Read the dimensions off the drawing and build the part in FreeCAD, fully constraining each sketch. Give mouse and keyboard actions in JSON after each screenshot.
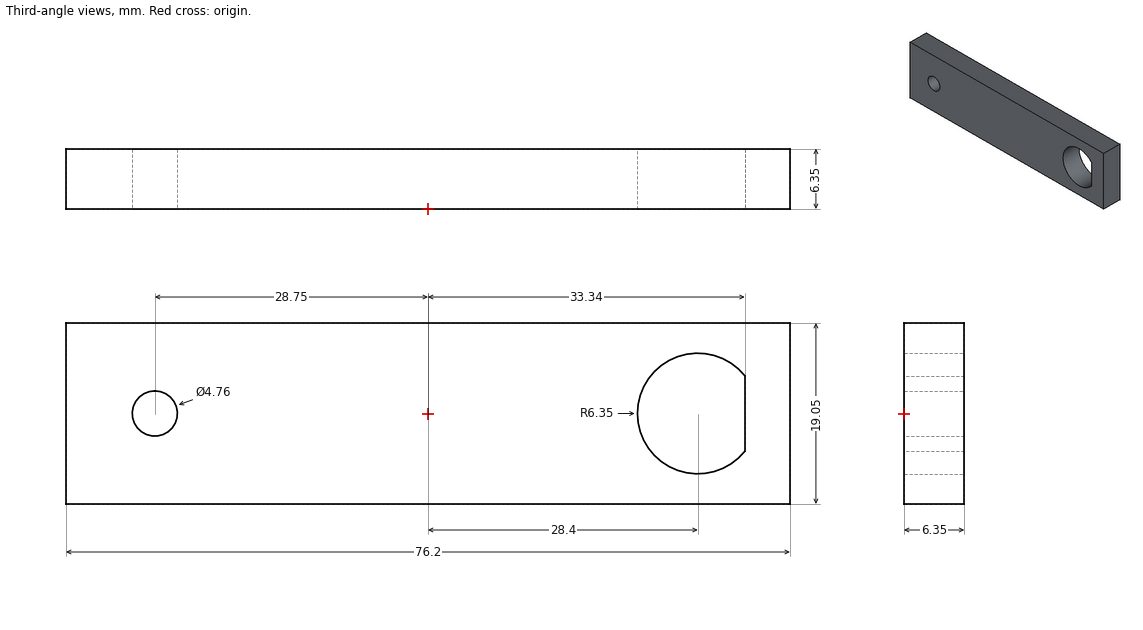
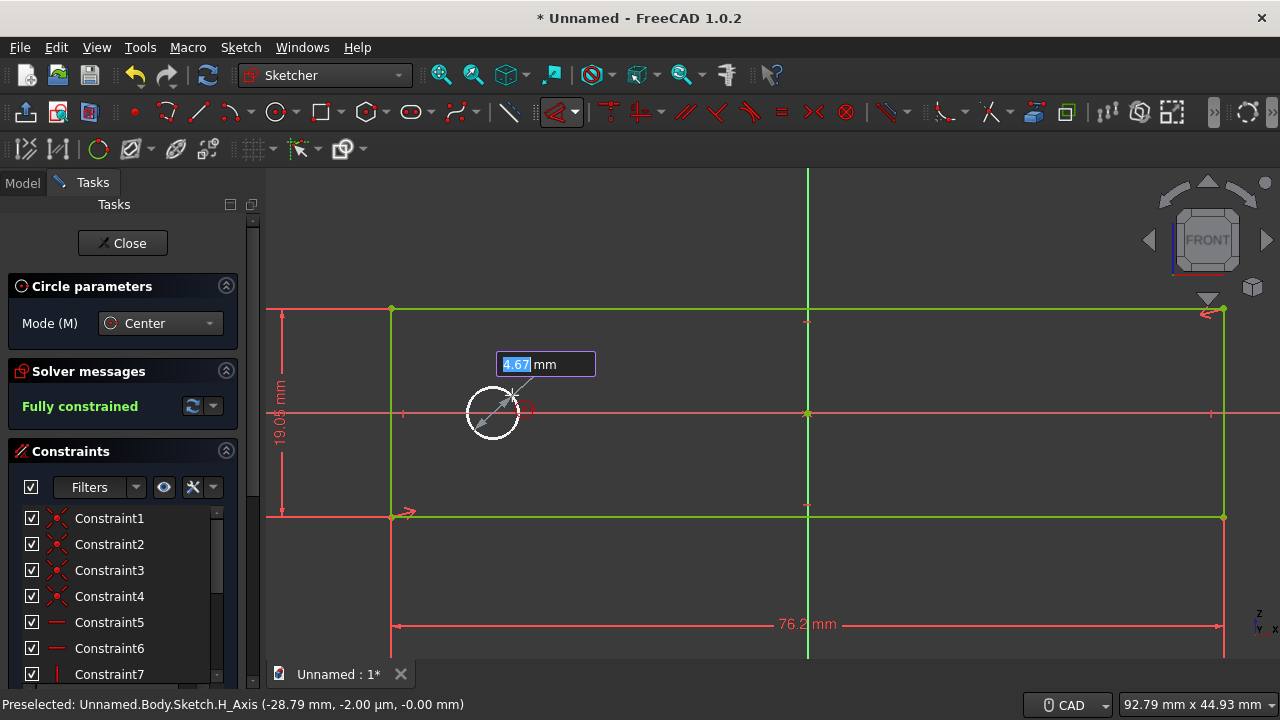
{"action": "type", "text": "4.76"}
{"action": "key", "text": "Return"}
{"action": "key", "text": "Escape"}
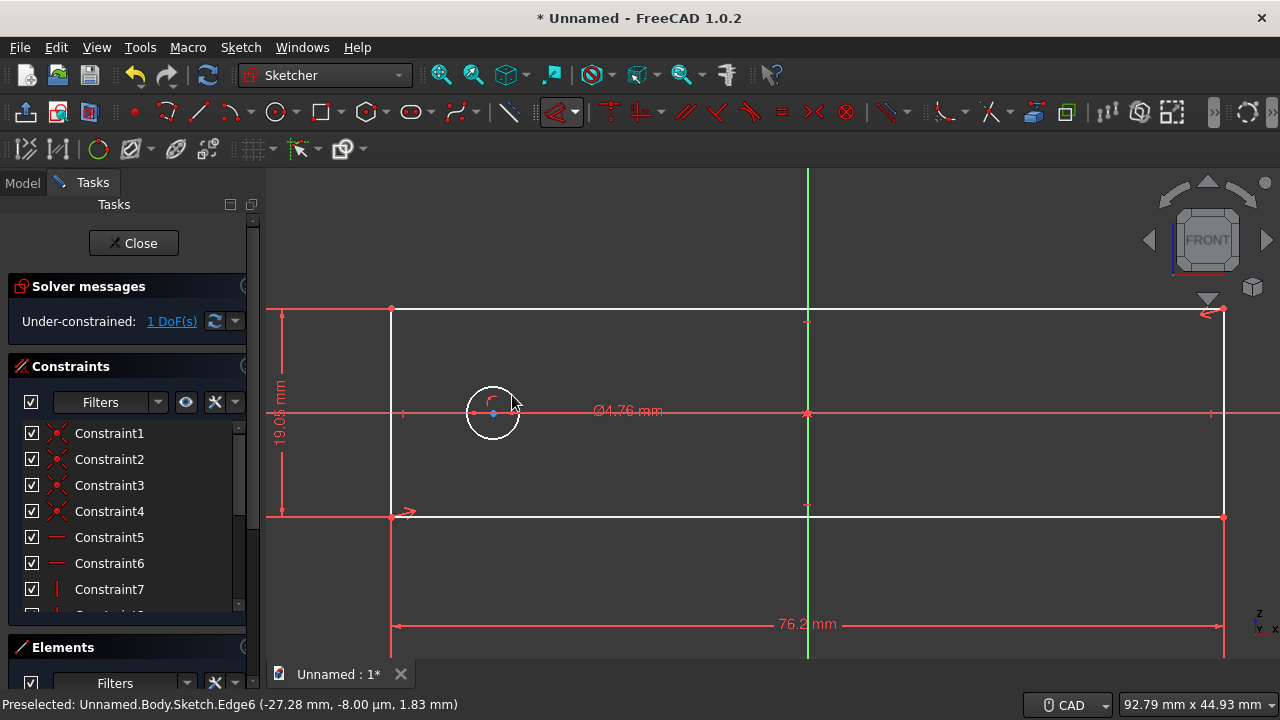
{"action": "left_click", "coordinate": [493, 413]}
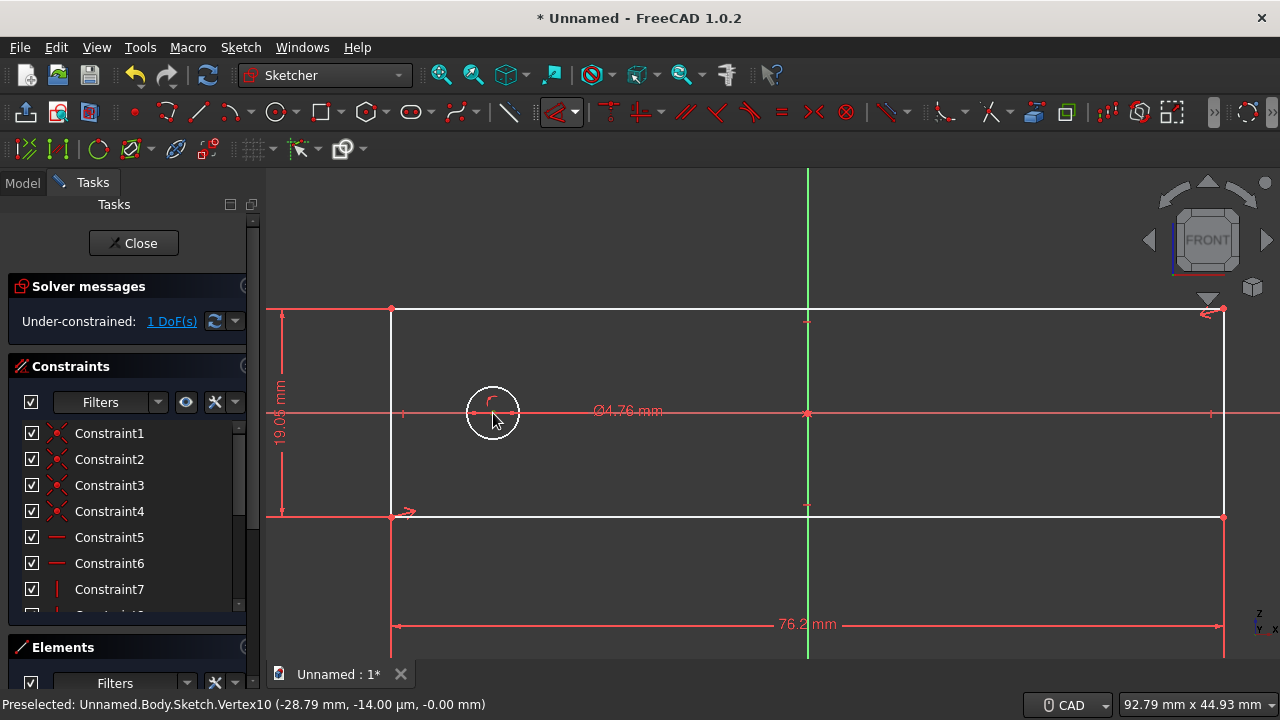
{"action": "left_click", "coordinate": [578, 112]}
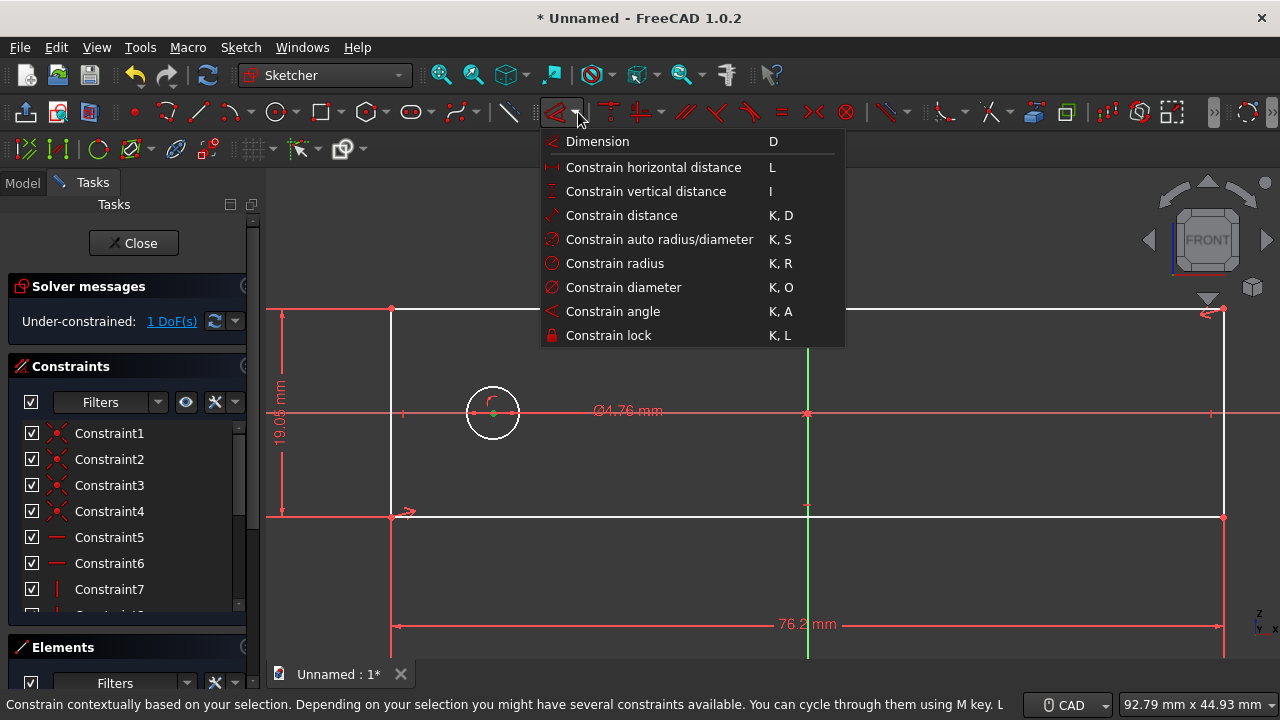
{"action": "left_click", "coordinate": [693, 167]}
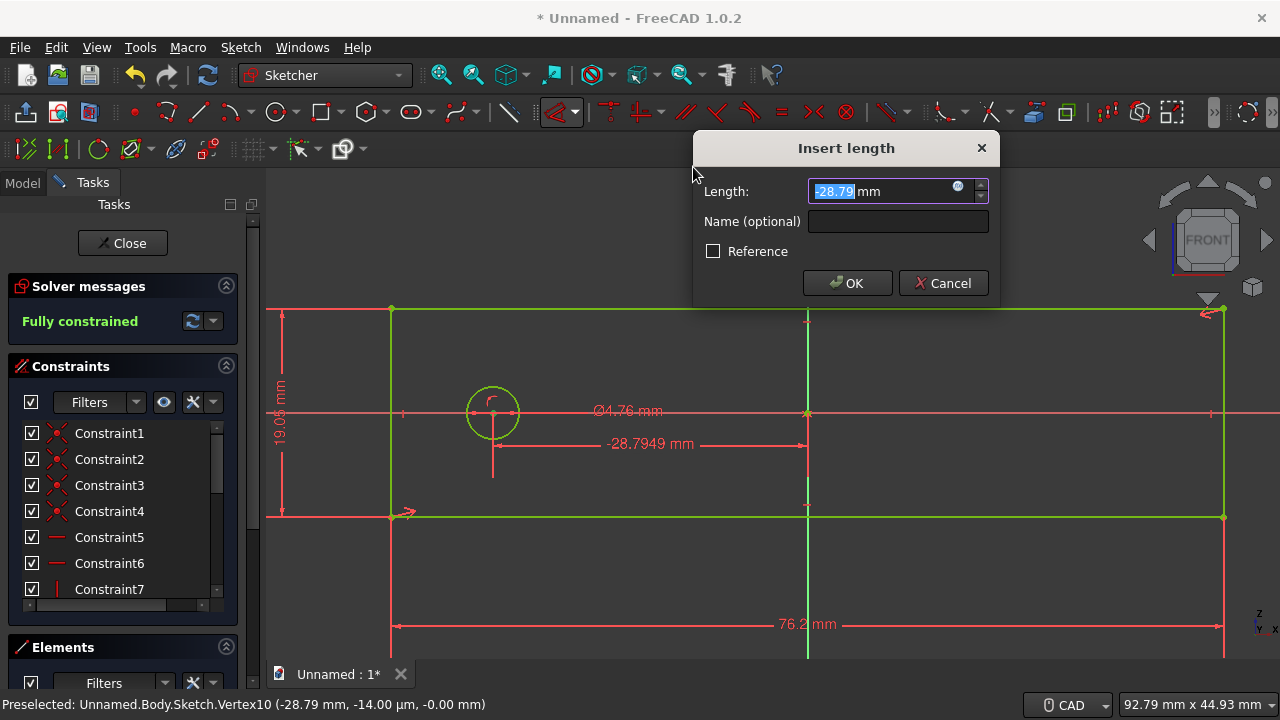
{"action": "type", "text": "-28.75"}
{"action": "key", "text": "Return"}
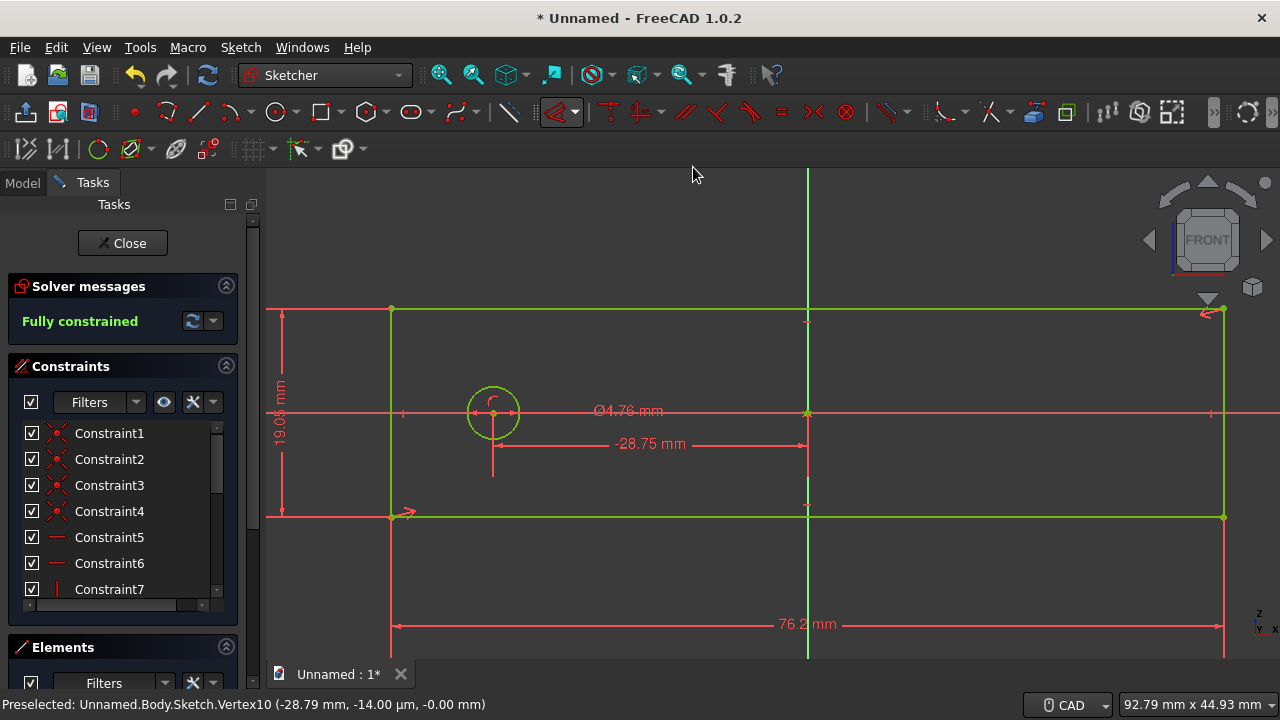
{"action": "left_click", "coordinate": [123, 243]}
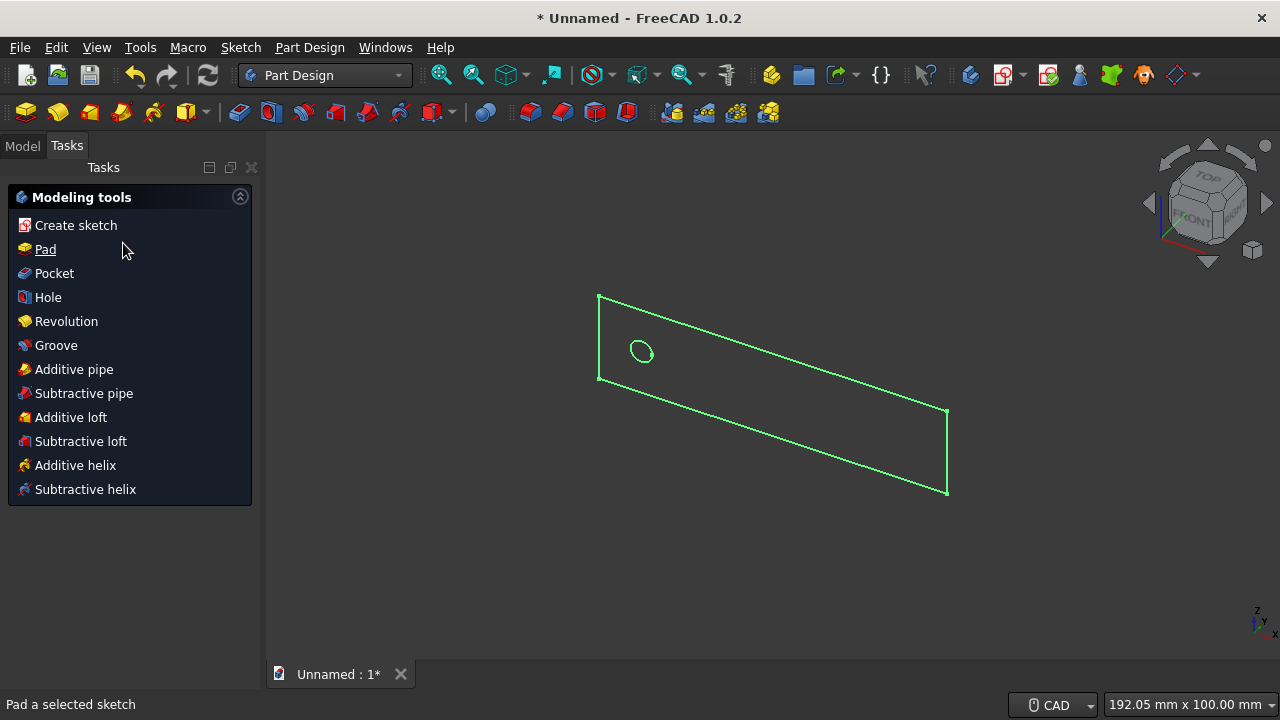
{"action": "left_click", "coordinate": [26, 112]}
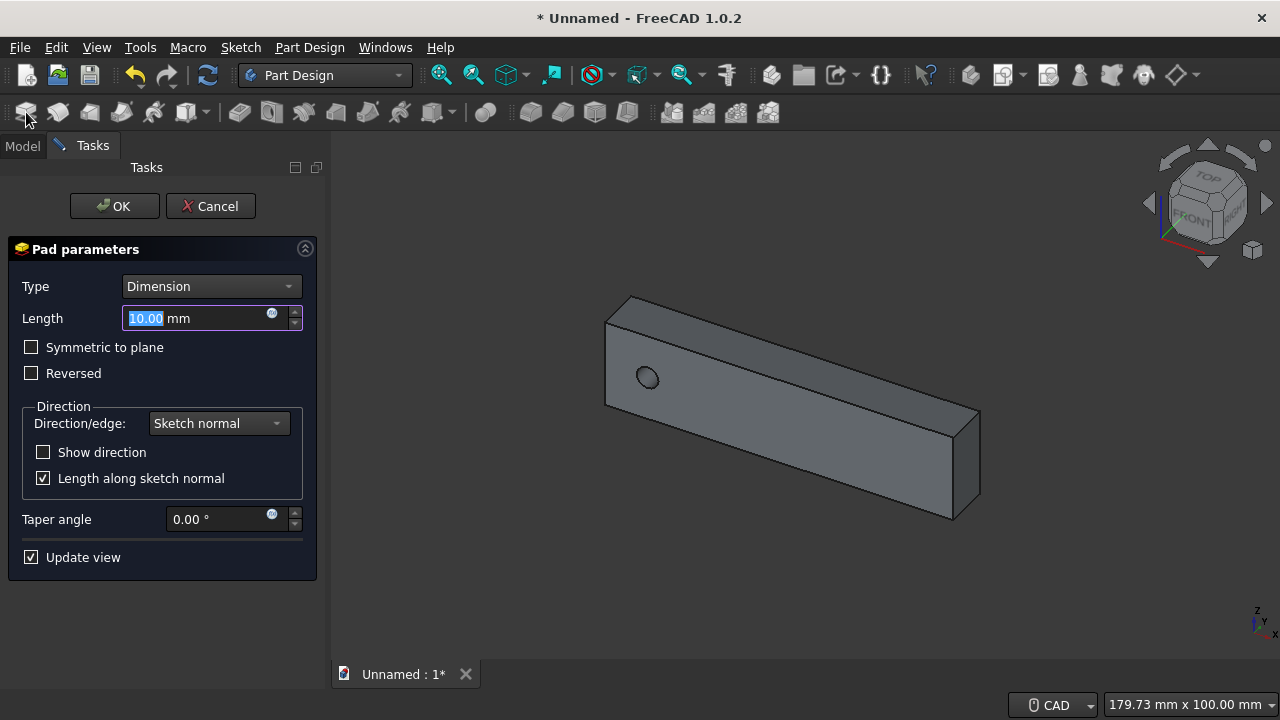
{"action": "type", "text": "6.35"}
{"action": "key", "text": "Tab"}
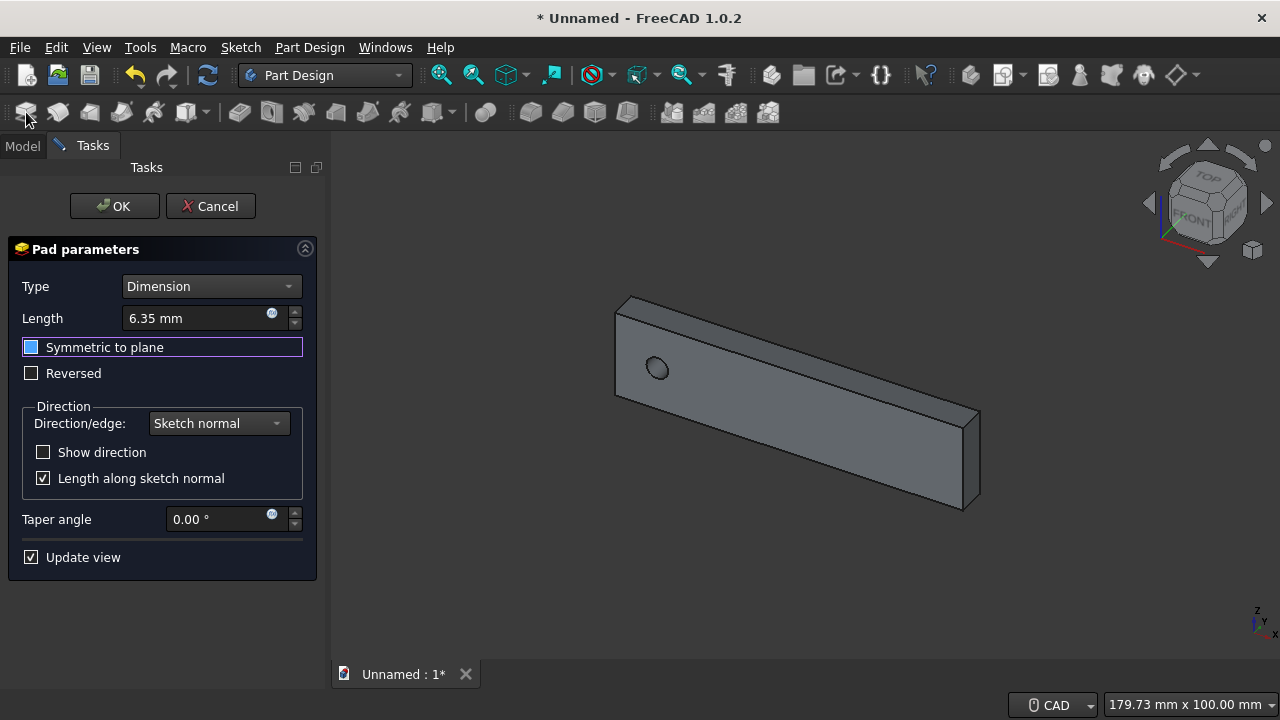
{"action": "left_click", "coordinate": [30, 373]}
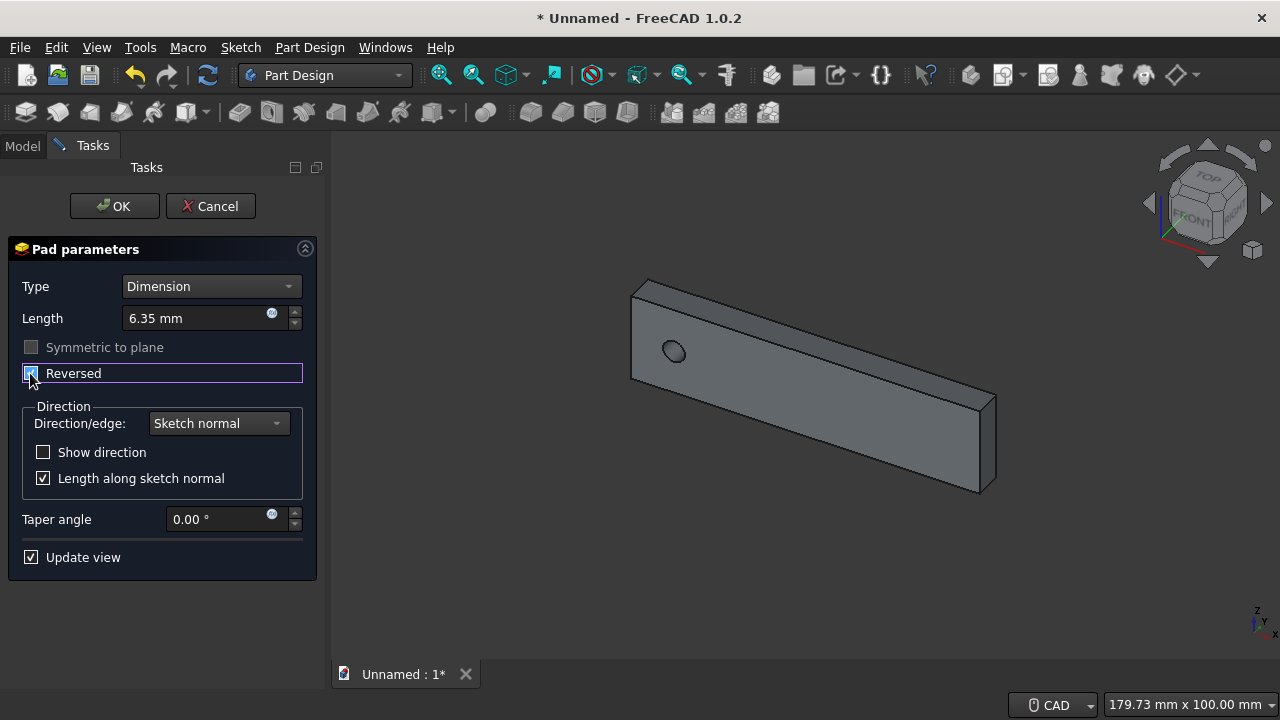
{"action": "left_click", "coordinate": [115, 206]}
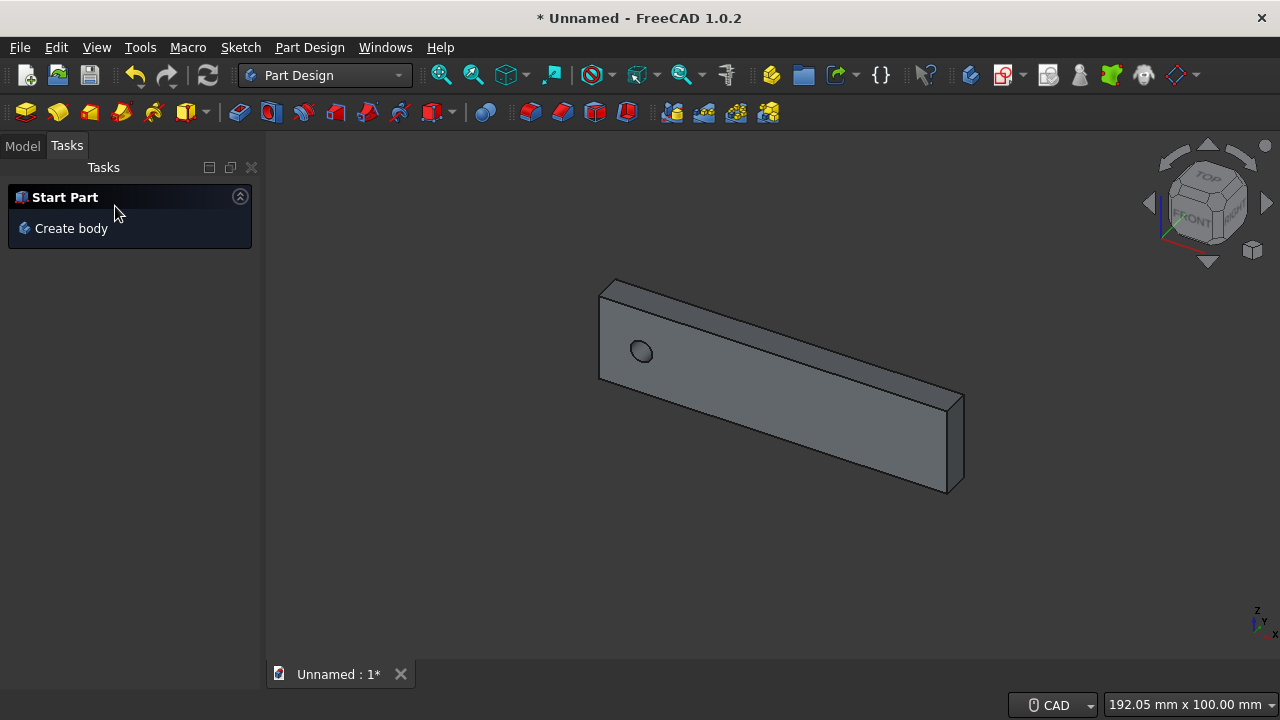
{"action": "key", "text": "v f"}